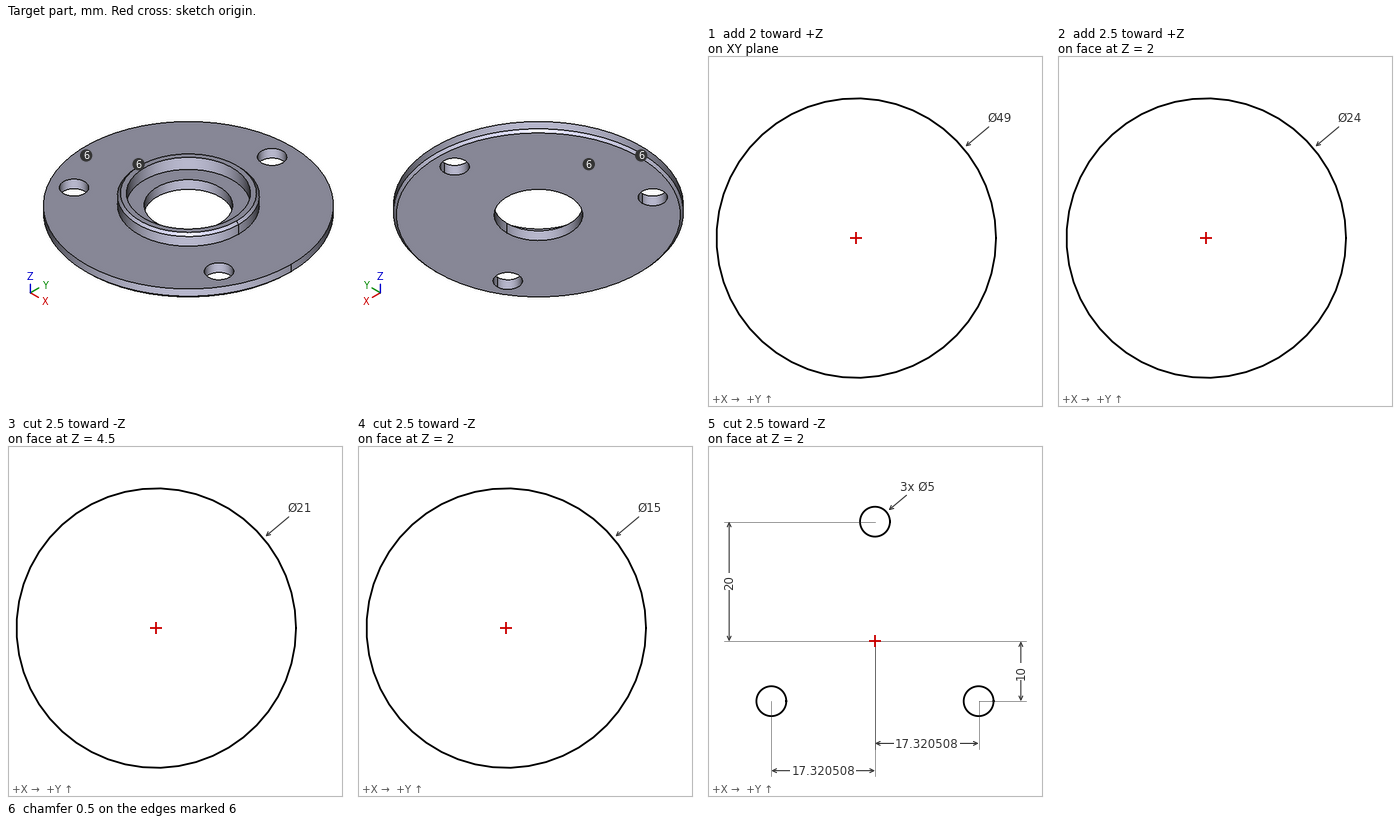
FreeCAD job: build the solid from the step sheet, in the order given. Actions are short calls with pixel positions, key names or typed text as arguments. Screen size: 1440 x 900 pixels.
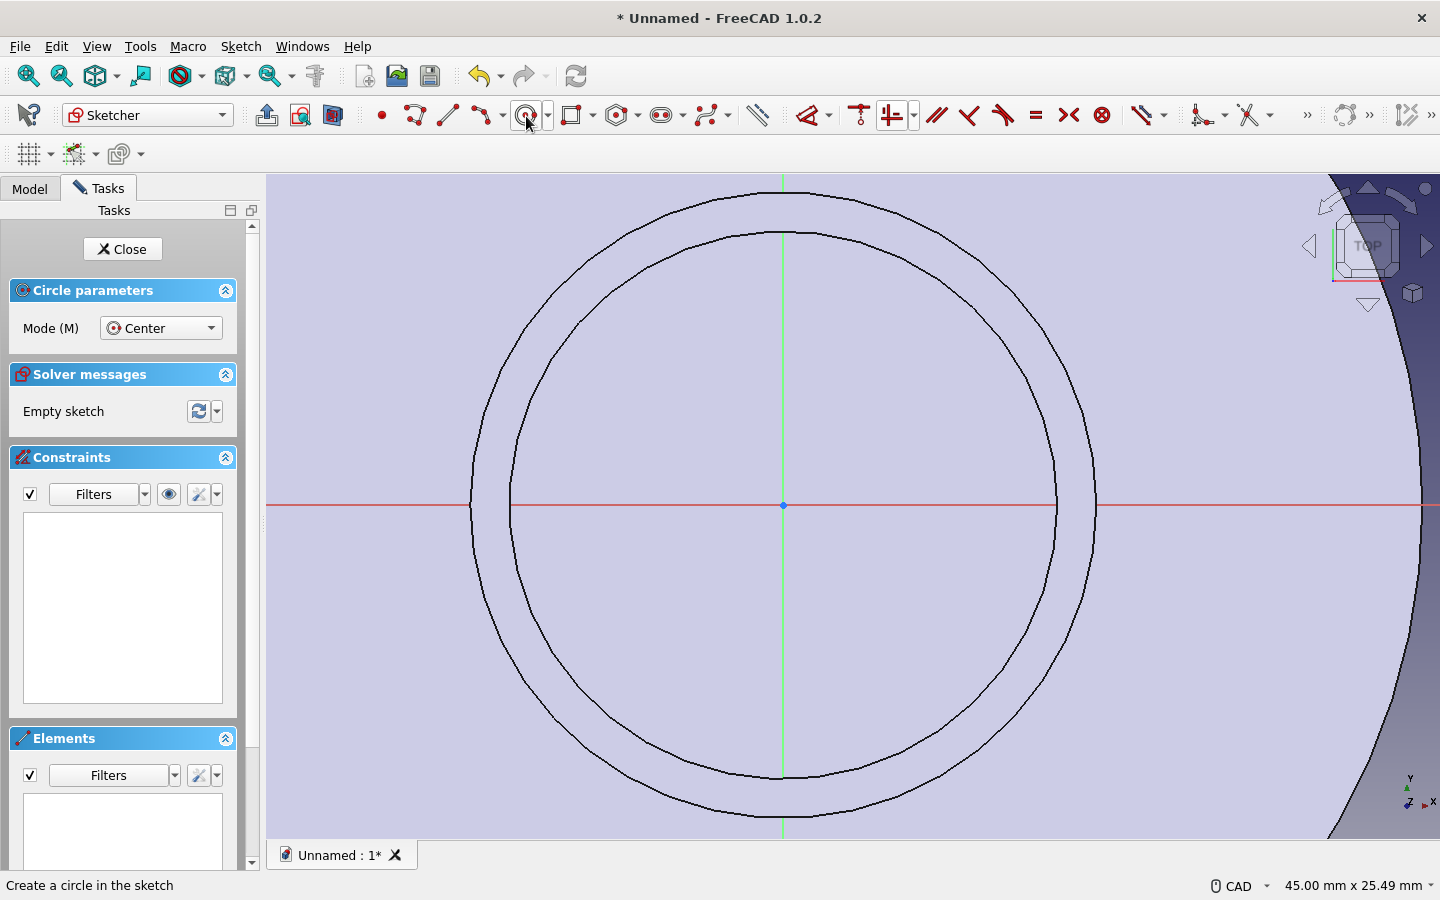
click(783, 505)
click(922, 367)
key(Escape)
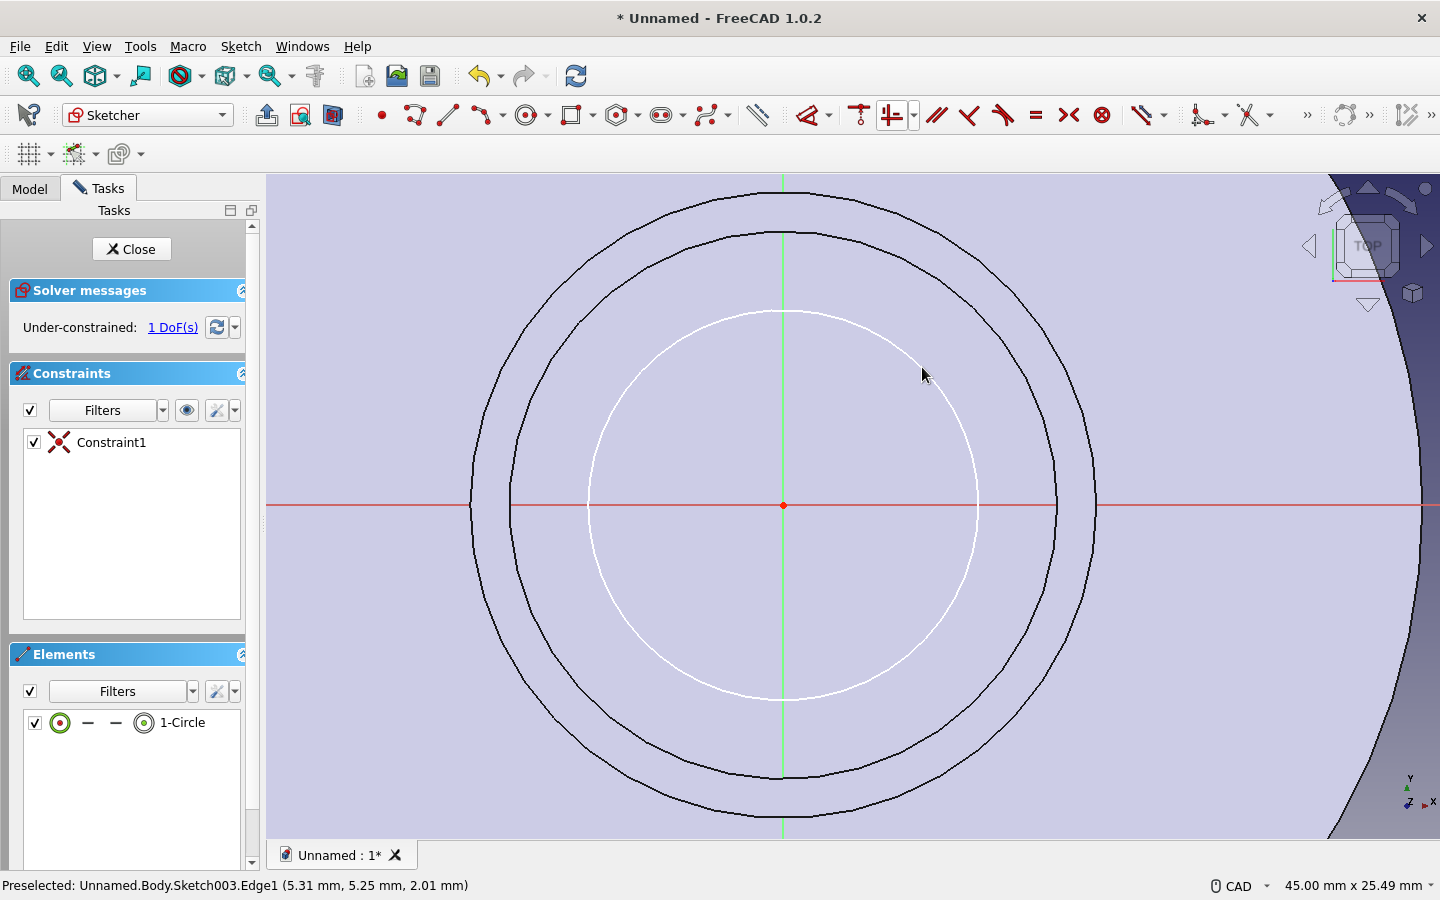
click(921, 367)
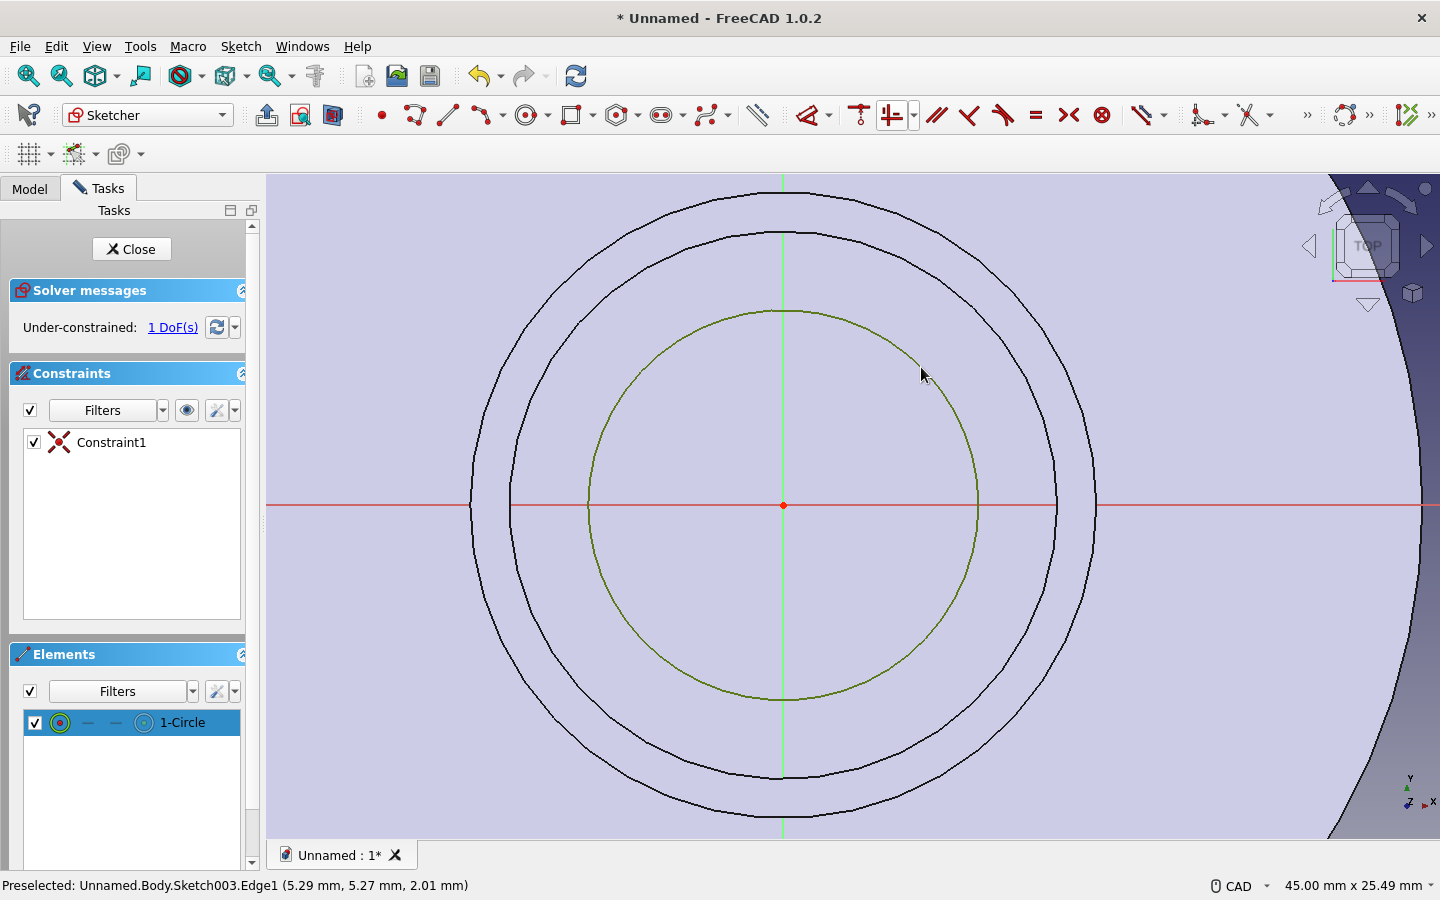
key(k)
key(o)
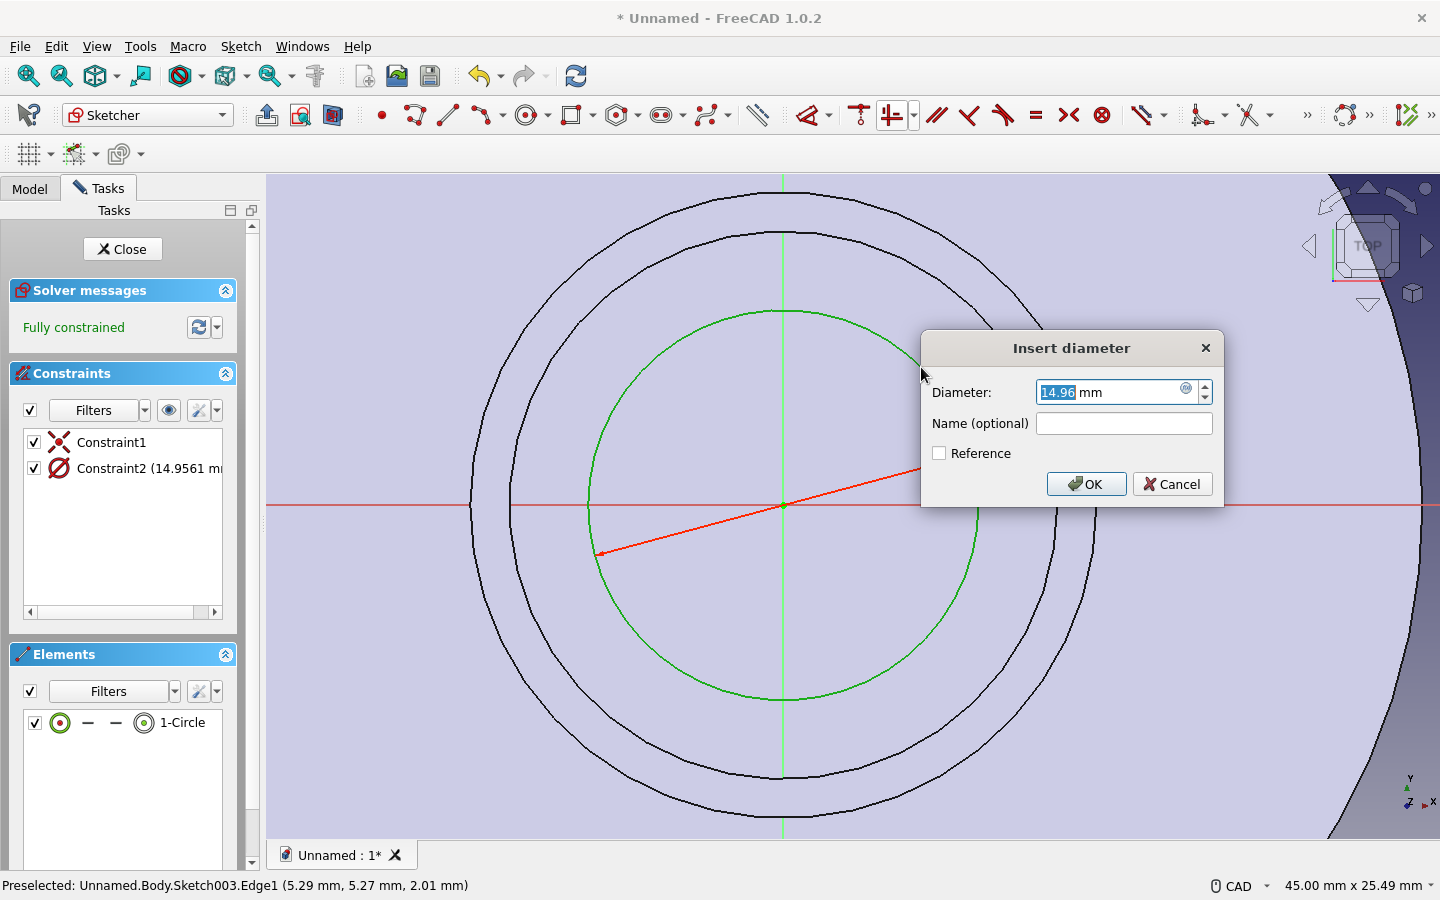
text(15)
key(Return)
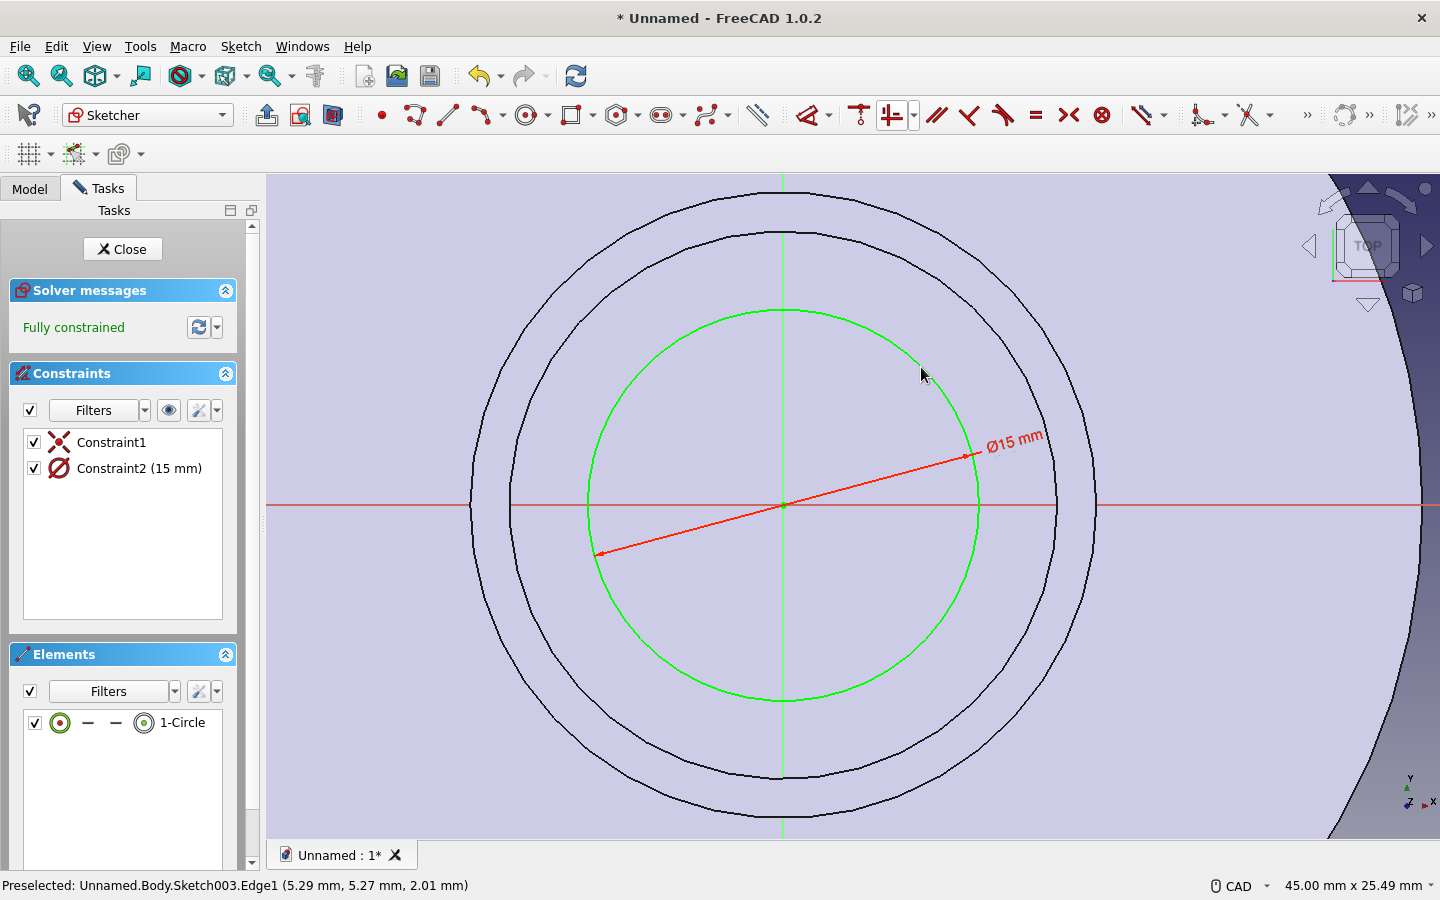
click(123, 249)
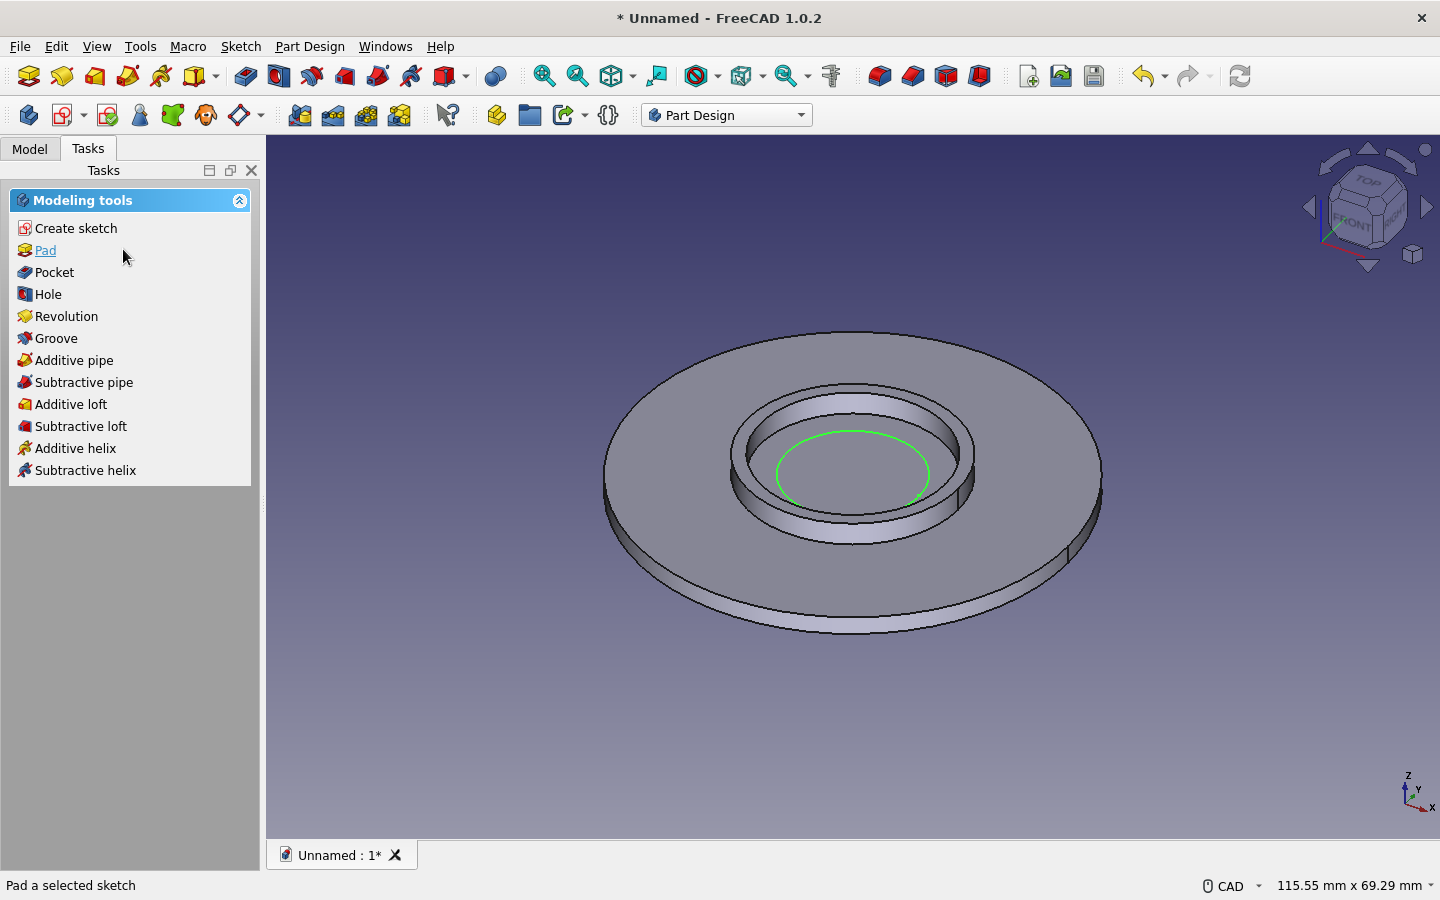
click(246, 76)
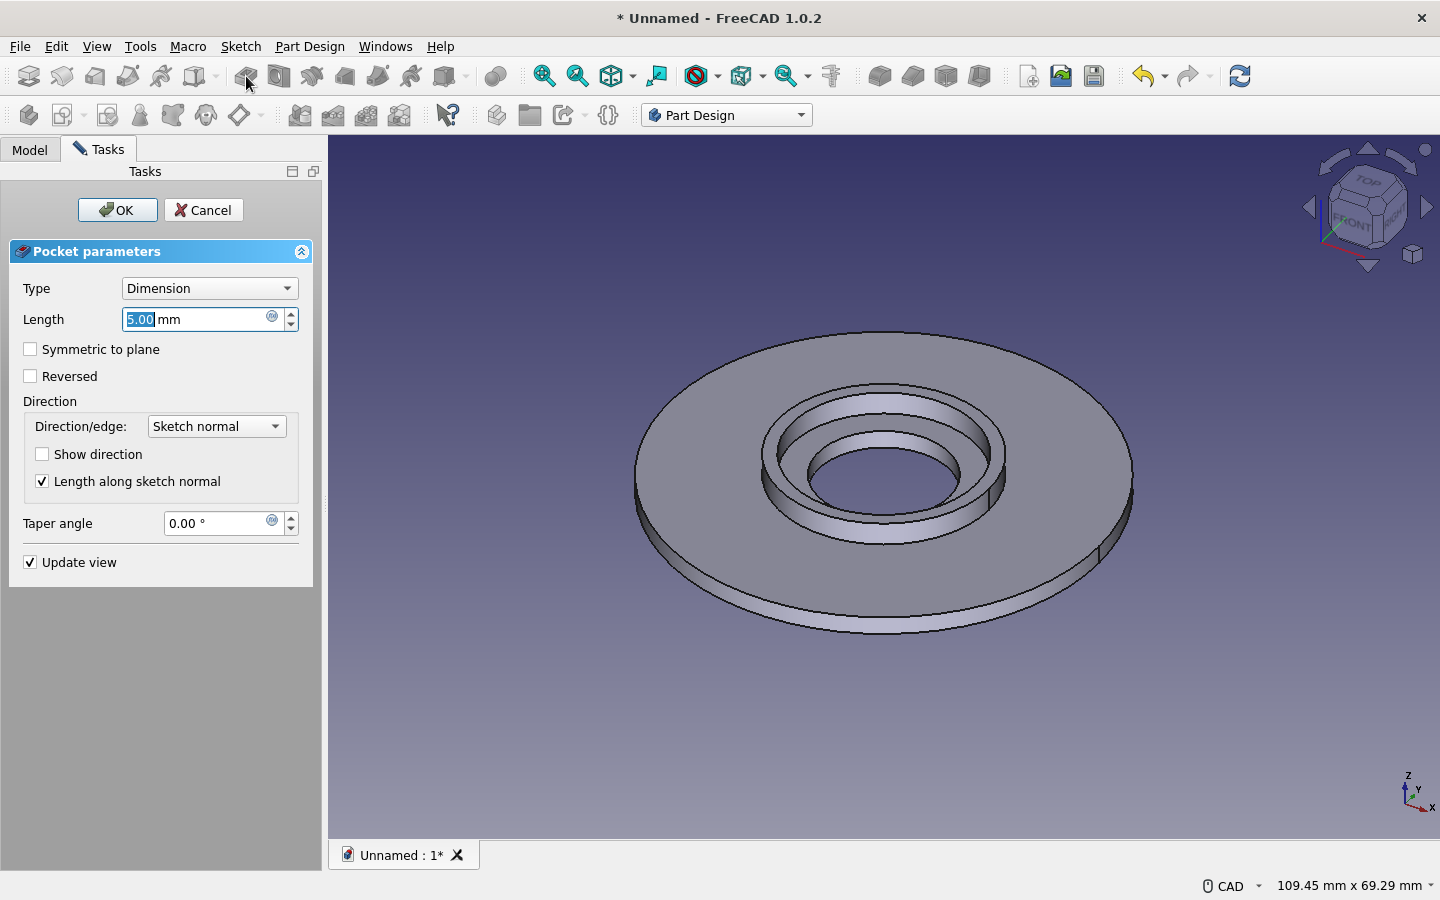
text(2.5)
key(Tab)